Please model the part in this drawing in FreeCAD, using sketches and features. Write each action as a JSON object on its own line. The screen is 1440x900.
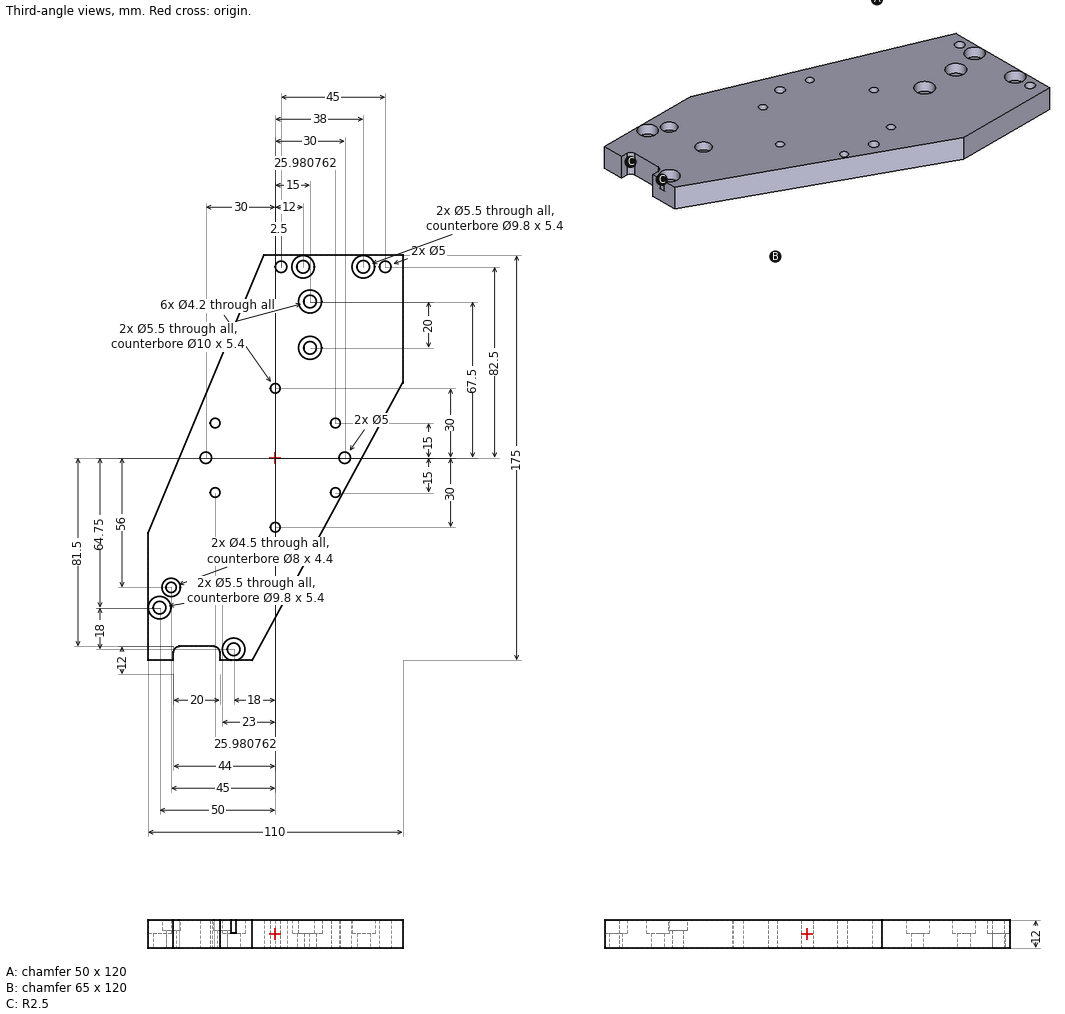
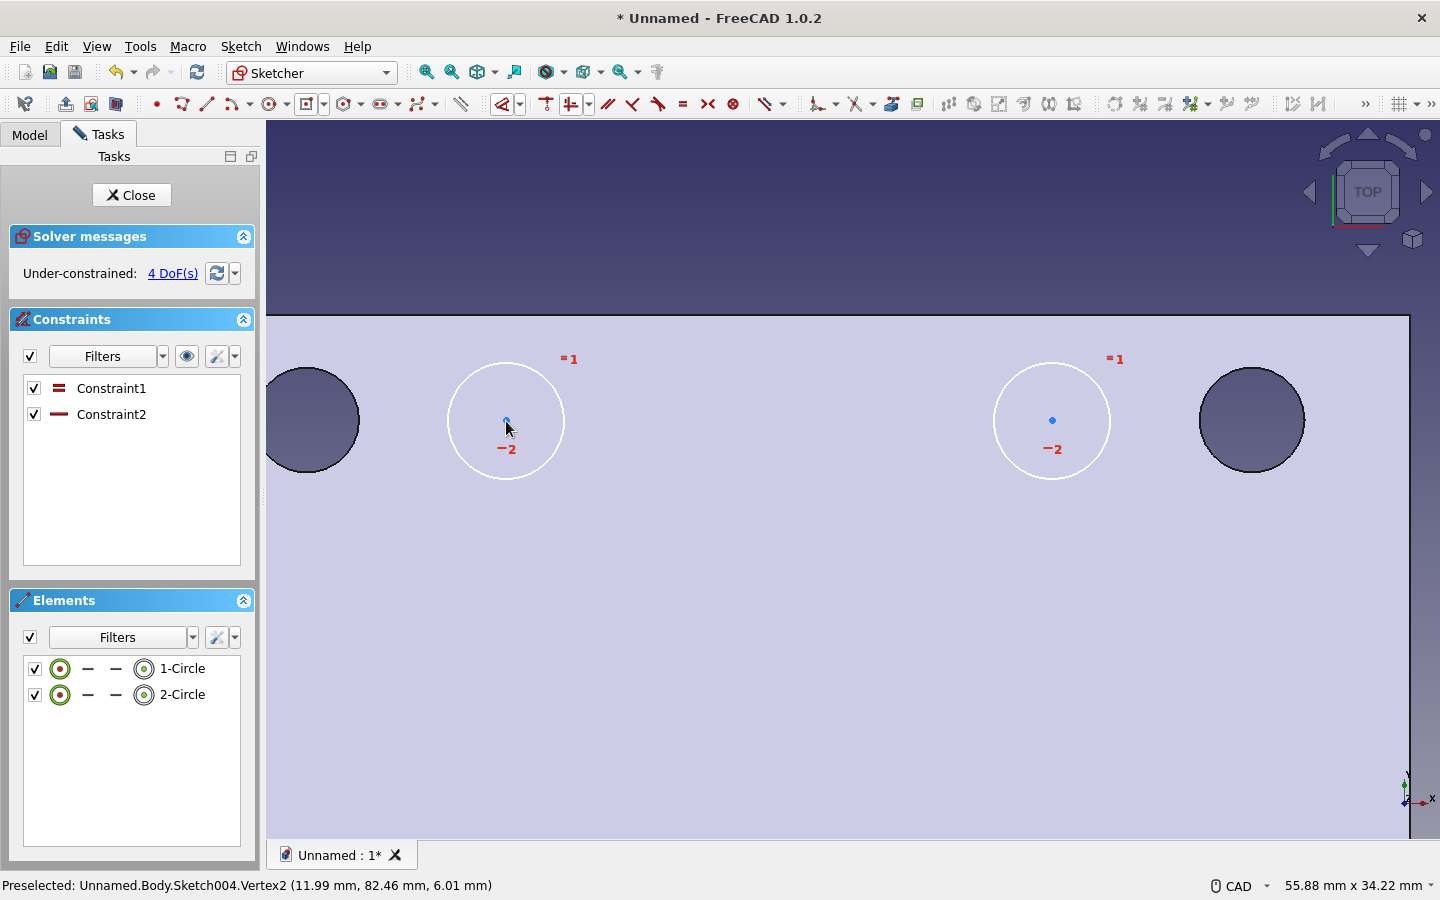
{"action": "left_click", "coordinate": [1093, 380]}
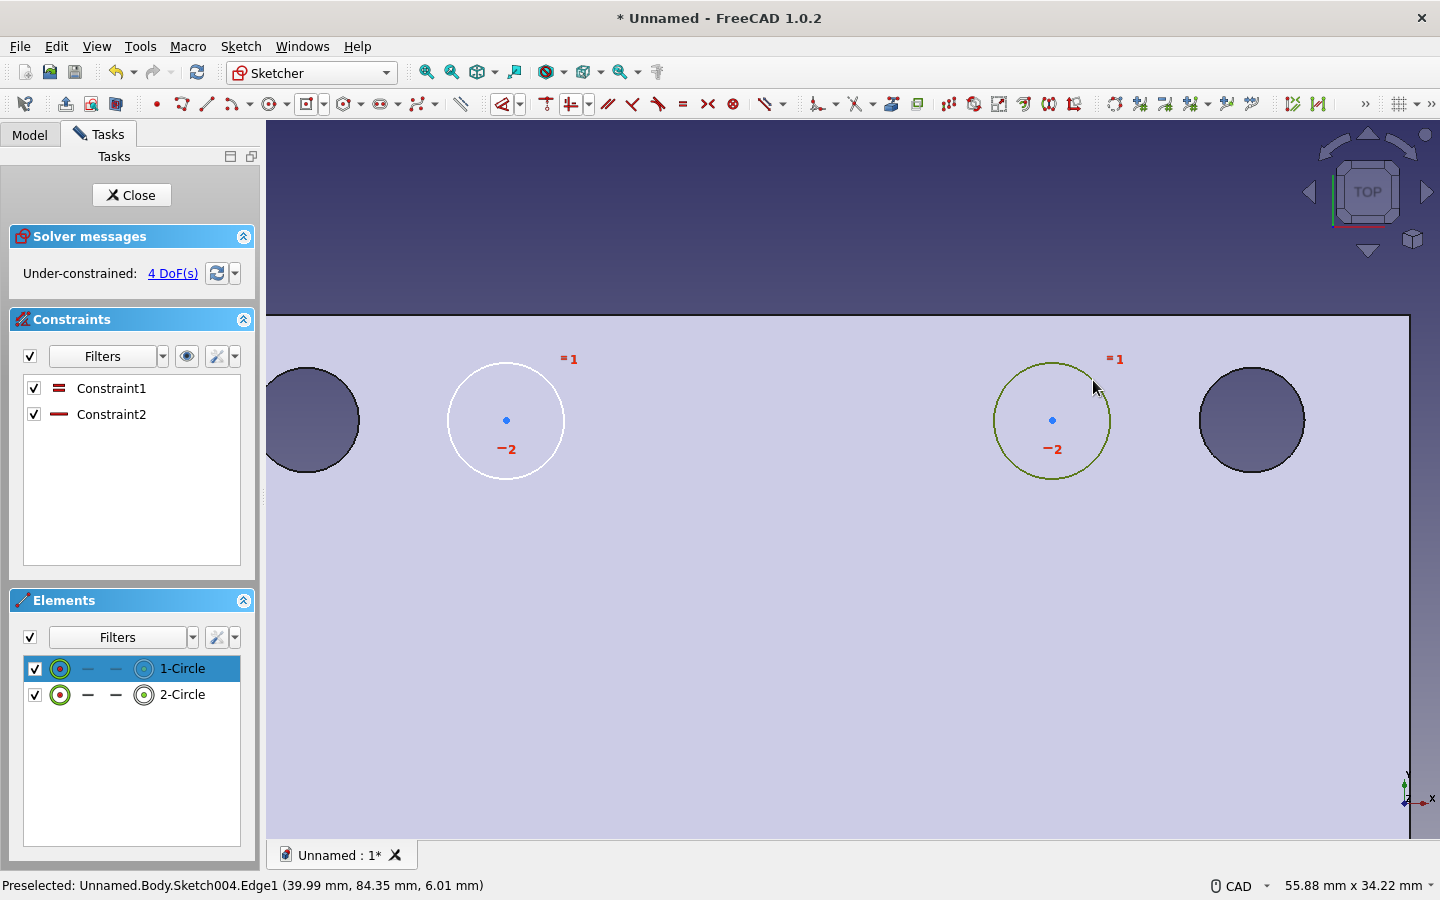
{"action": "key", "text": "k o"}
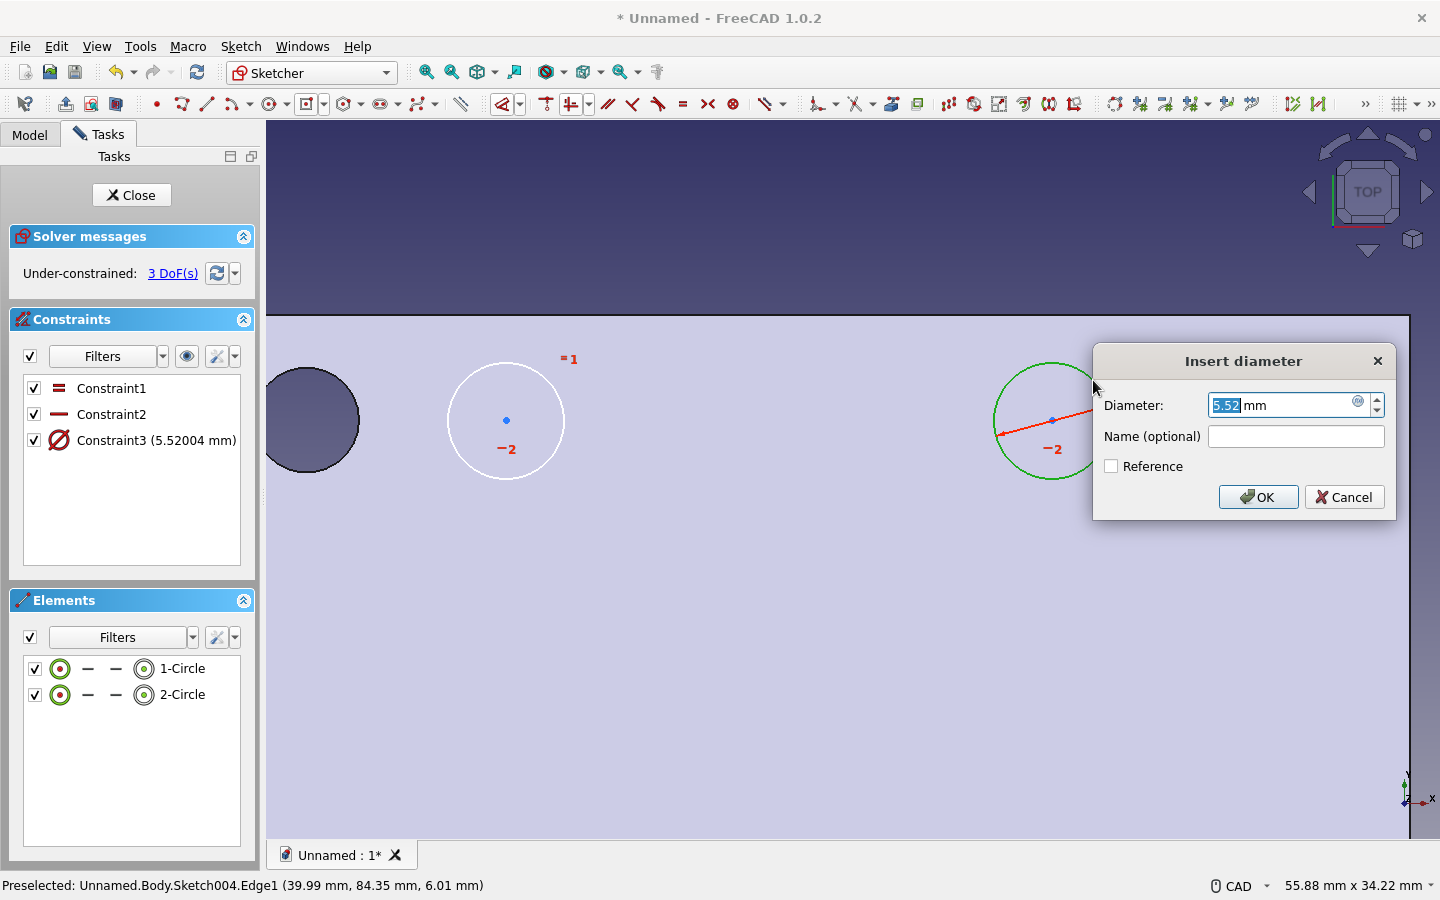
{"action": "type", "text": "5.5"}
{"action": "key", "text": "Return"}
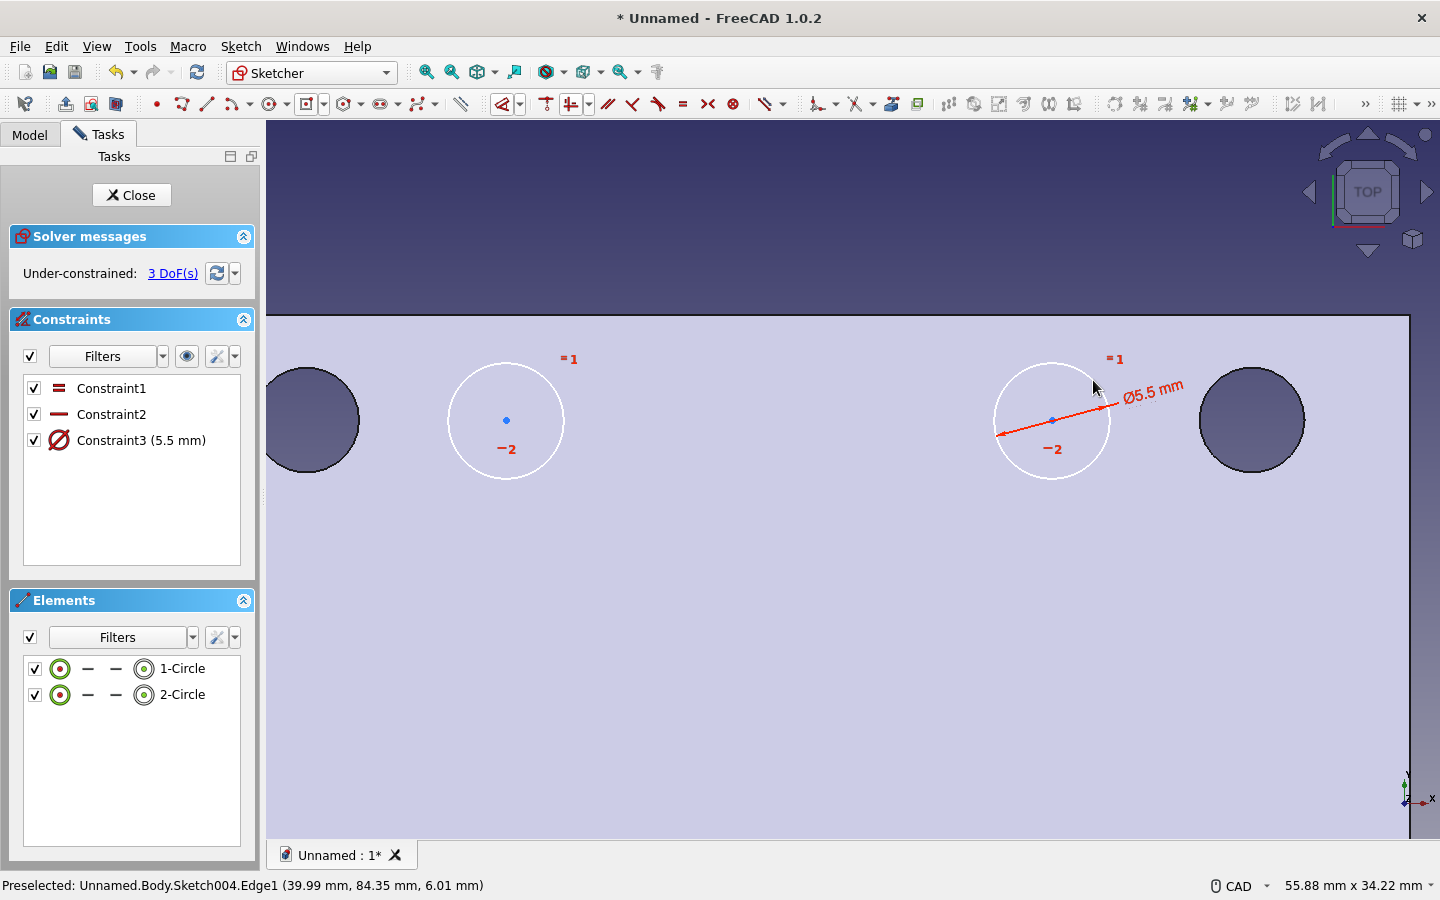
{"action": "left_click", "coordinate": [1052, 421]}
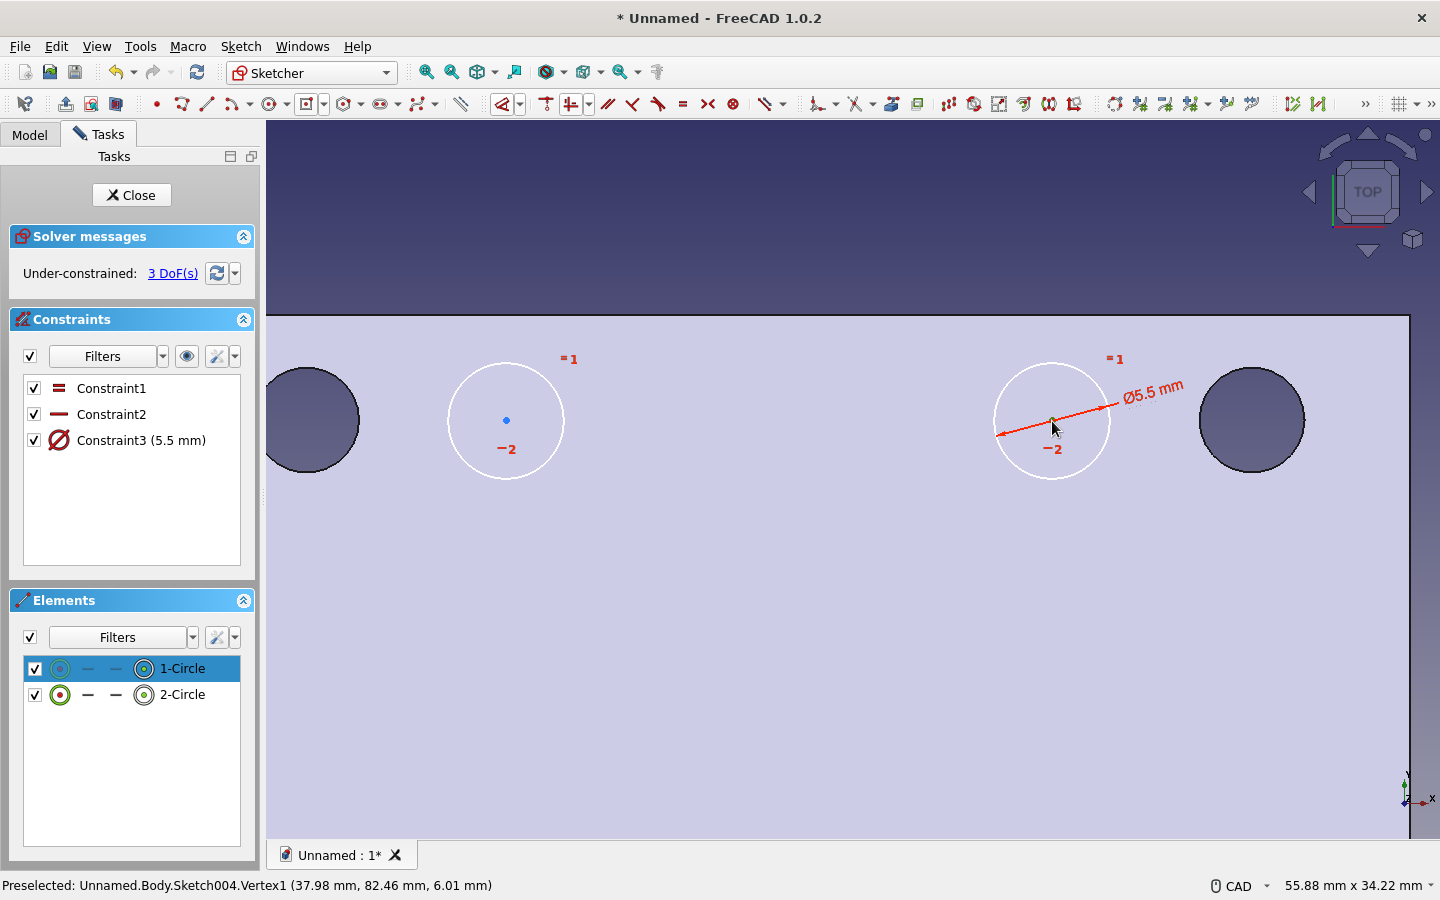
{"action": "key", "text": "l"}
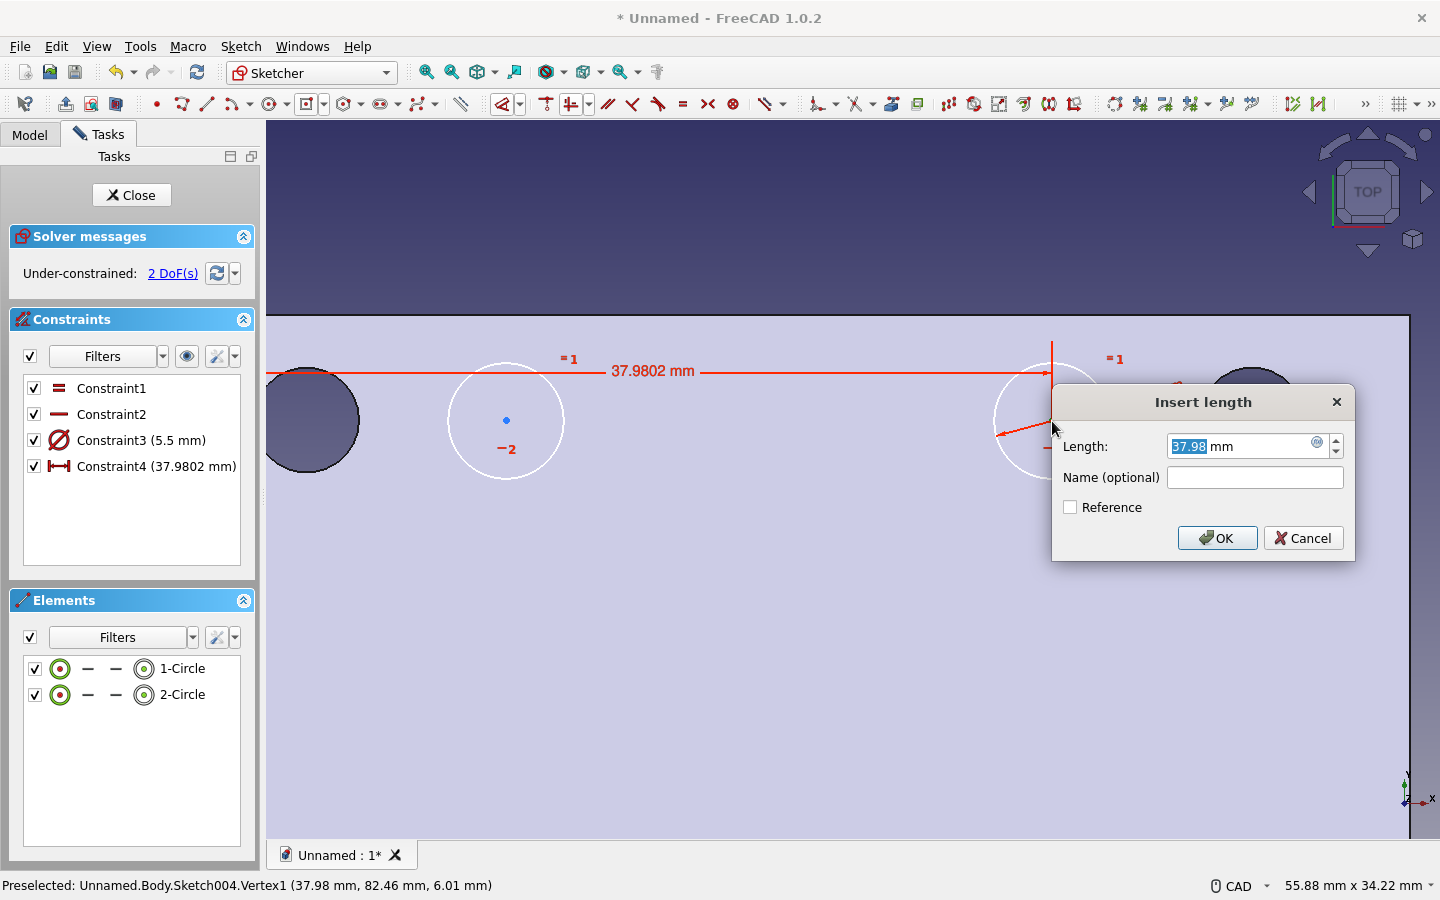
{"action": "type", "text": "38"}
{"action": "key", "text": "Return"}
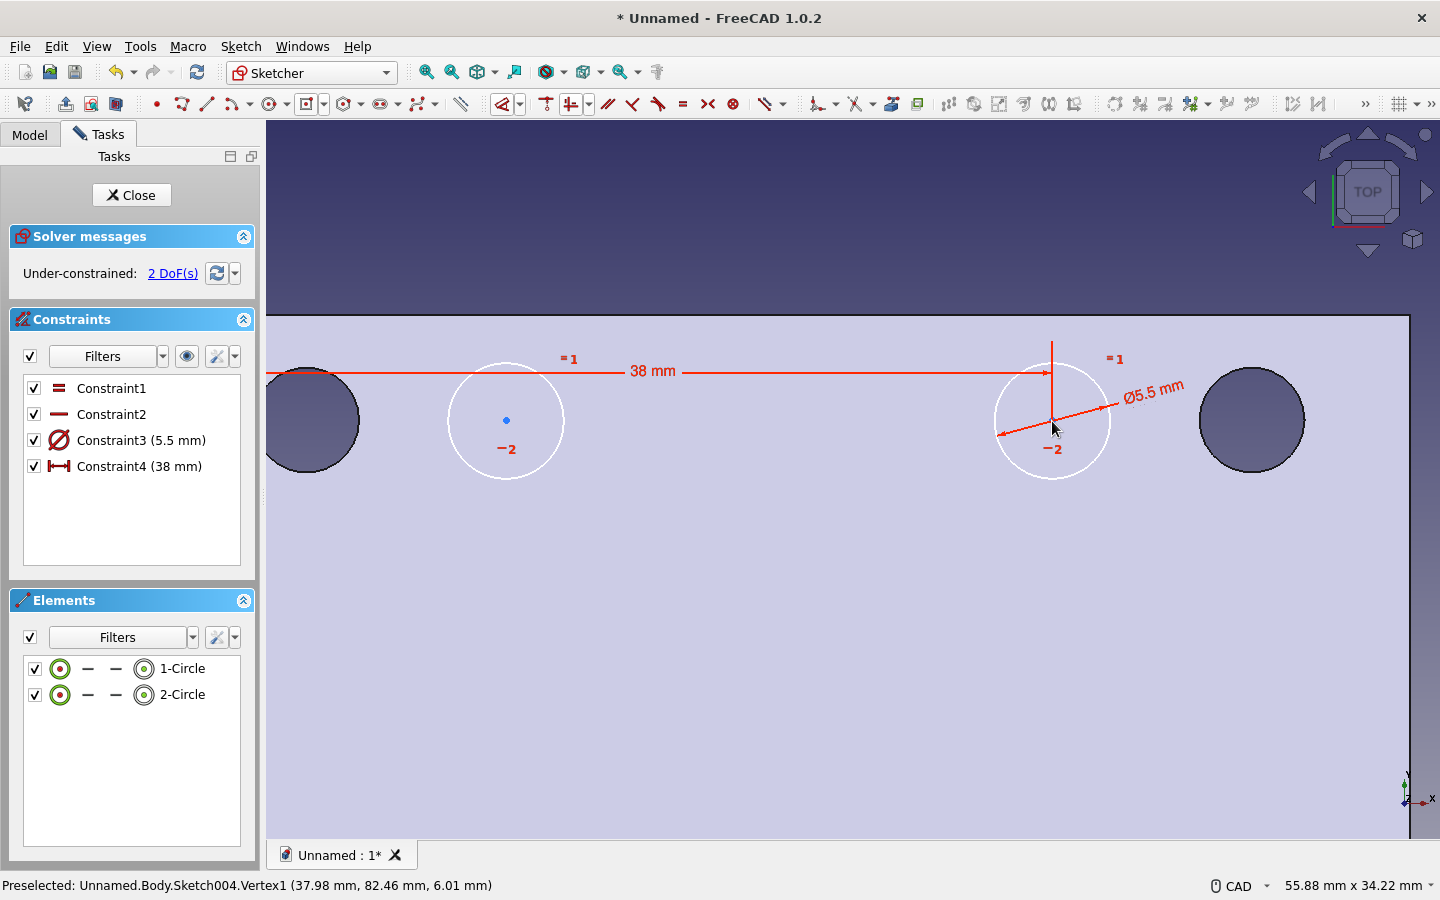
{"action": "left_click", "coordinate": [506, 421]}